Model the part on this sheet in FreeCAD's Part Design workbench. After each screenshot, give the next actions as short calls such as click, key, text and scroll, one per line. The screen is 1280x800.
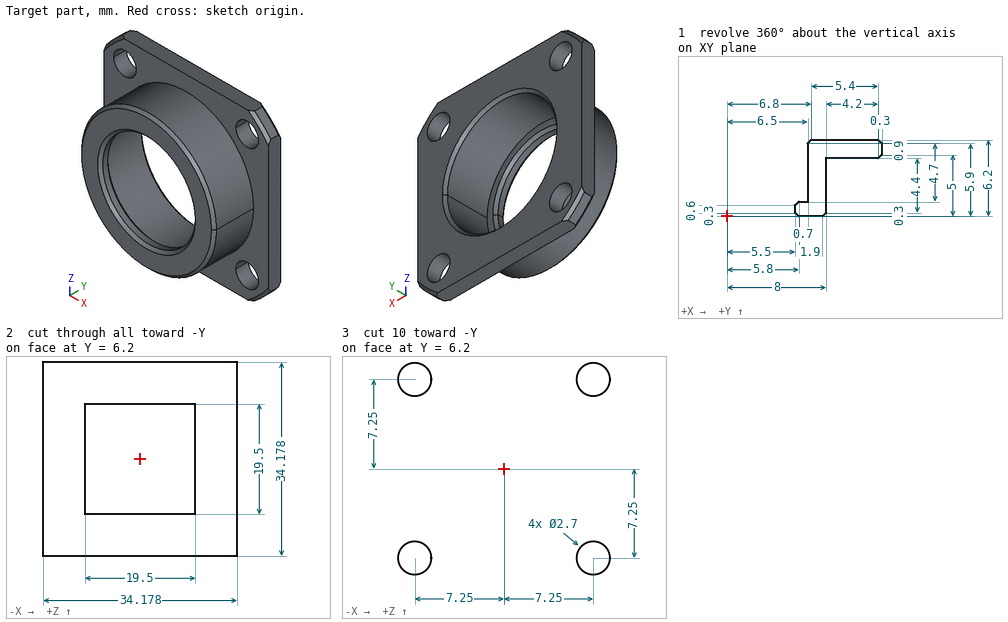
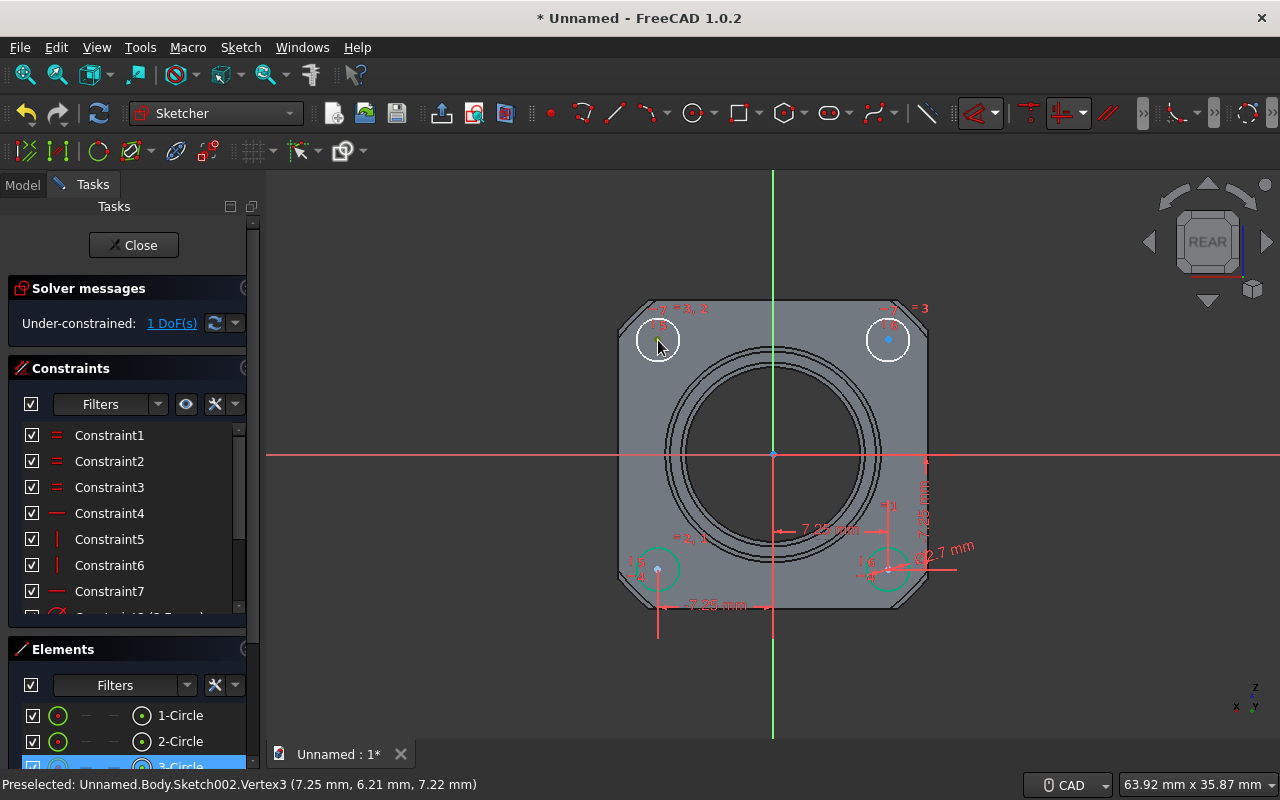
key(i)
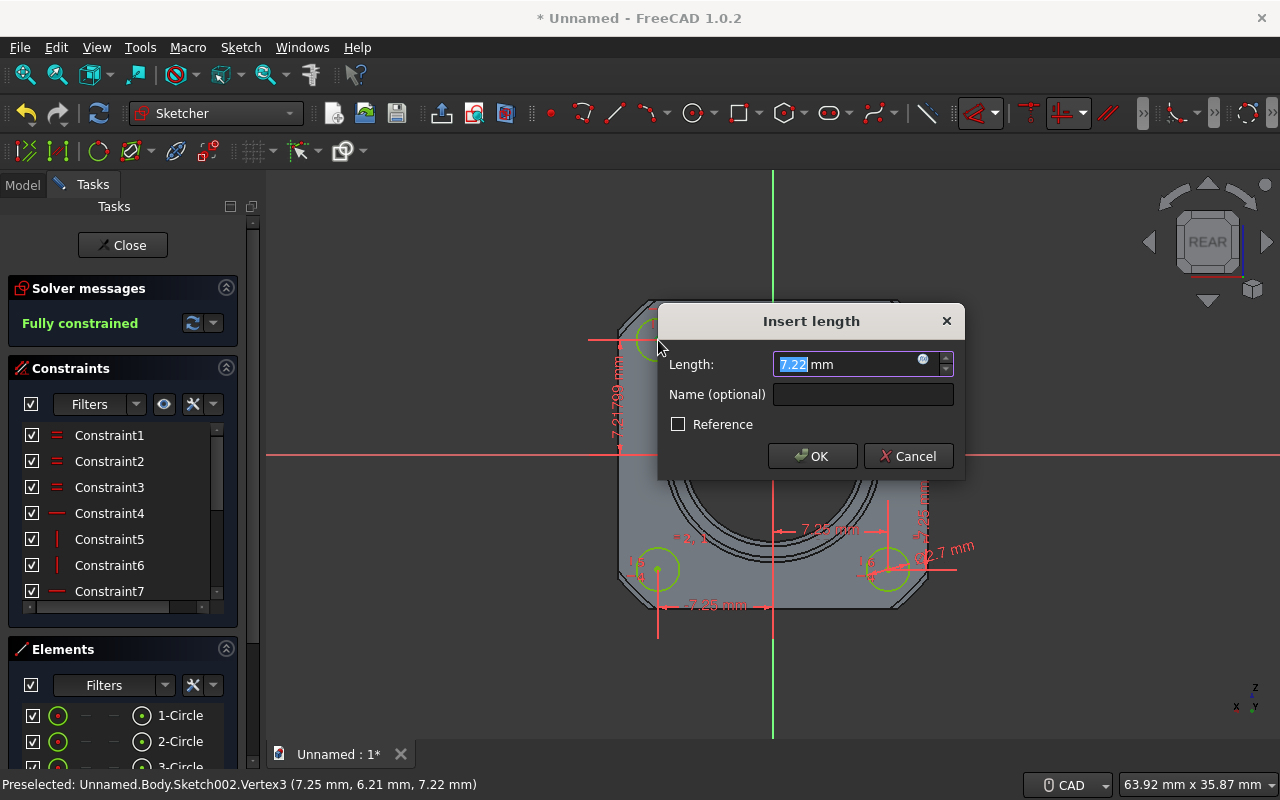
text(7.25)
key(Return)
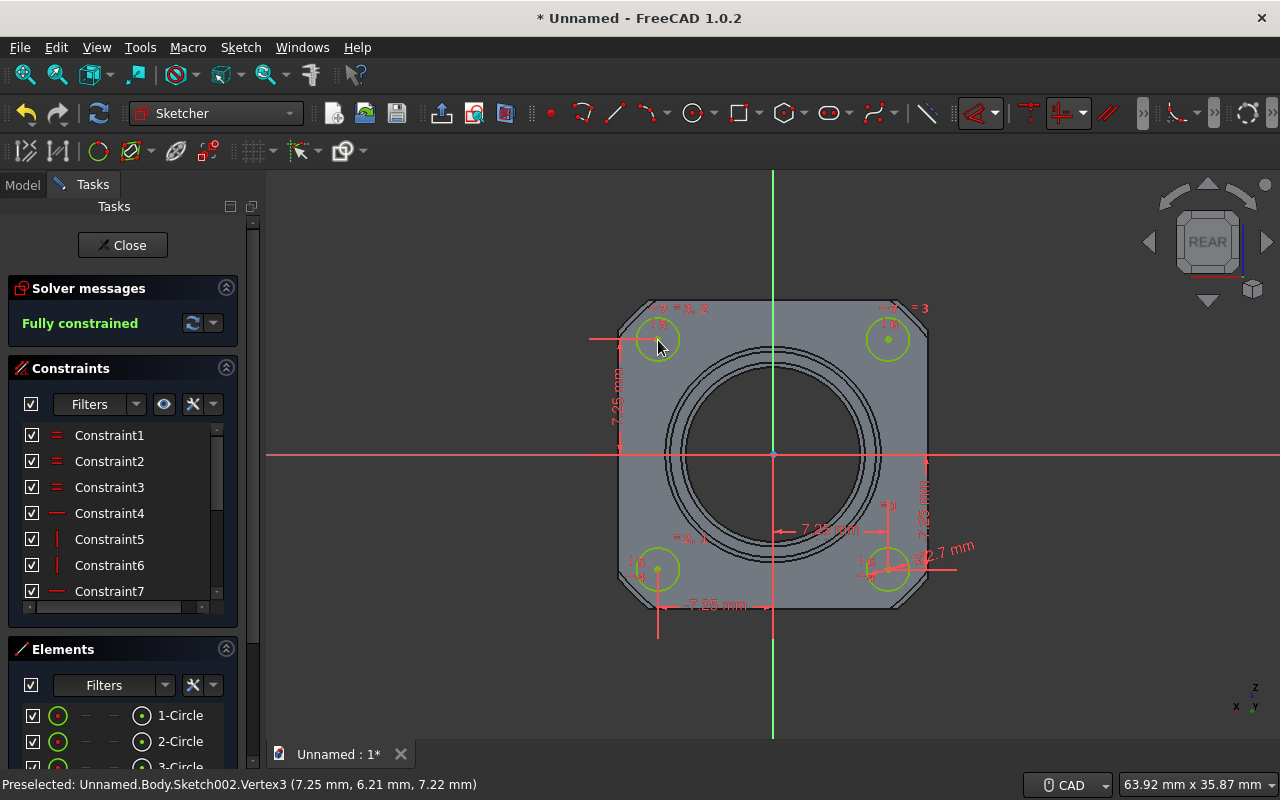
click(123, 245)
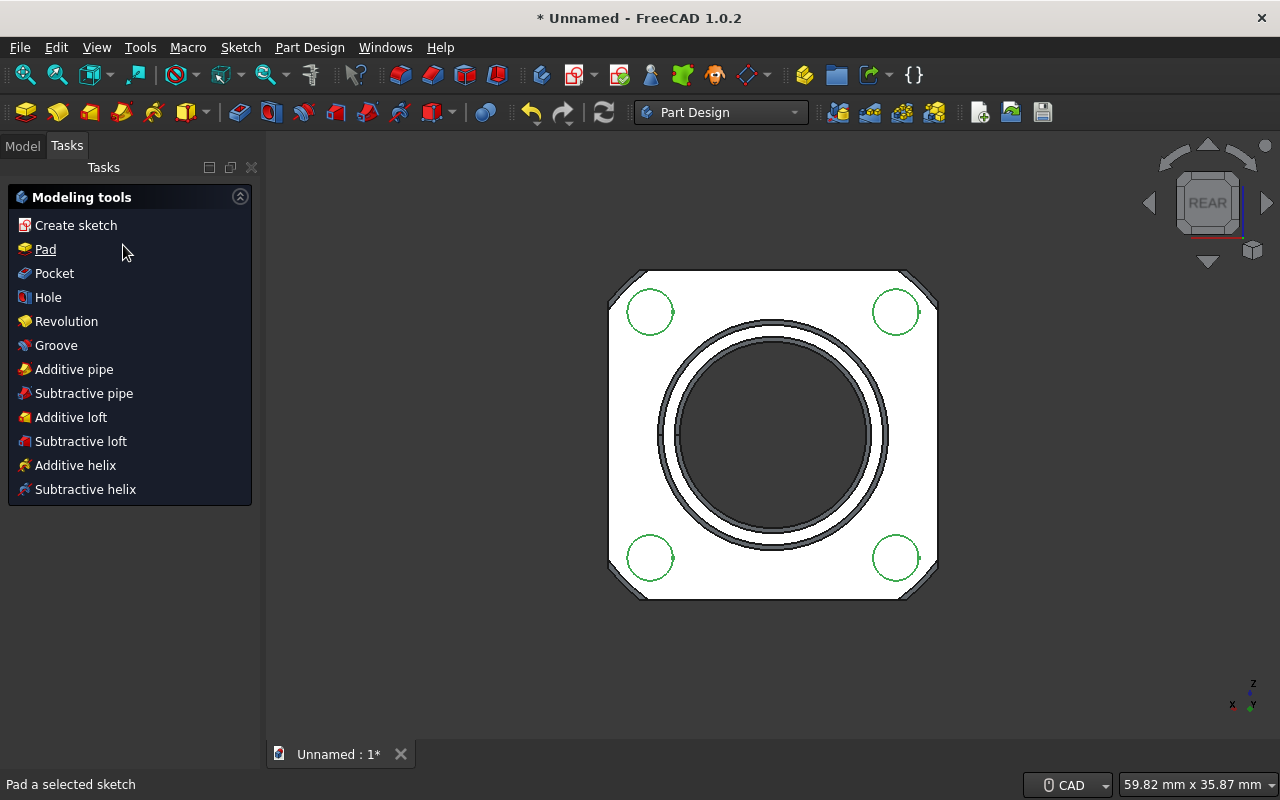
click(240, 112)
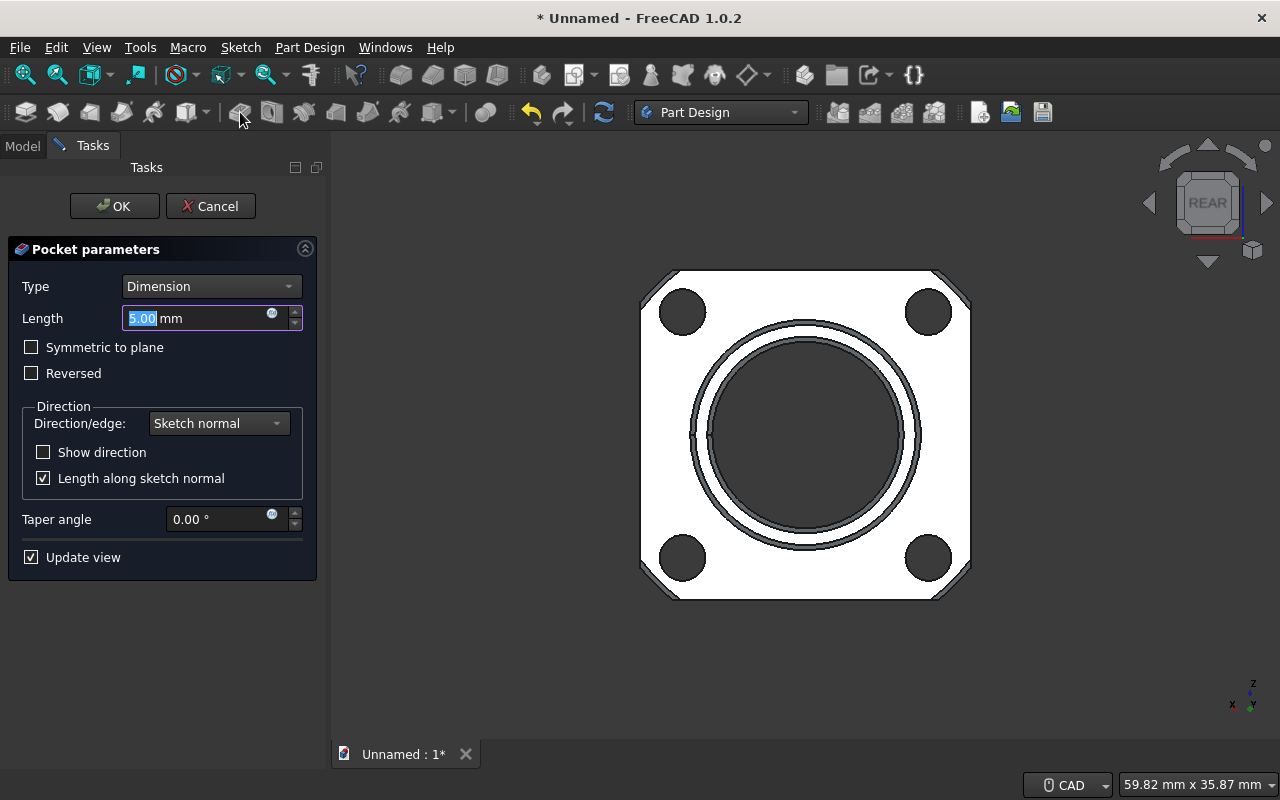
text(10)
key(Tab)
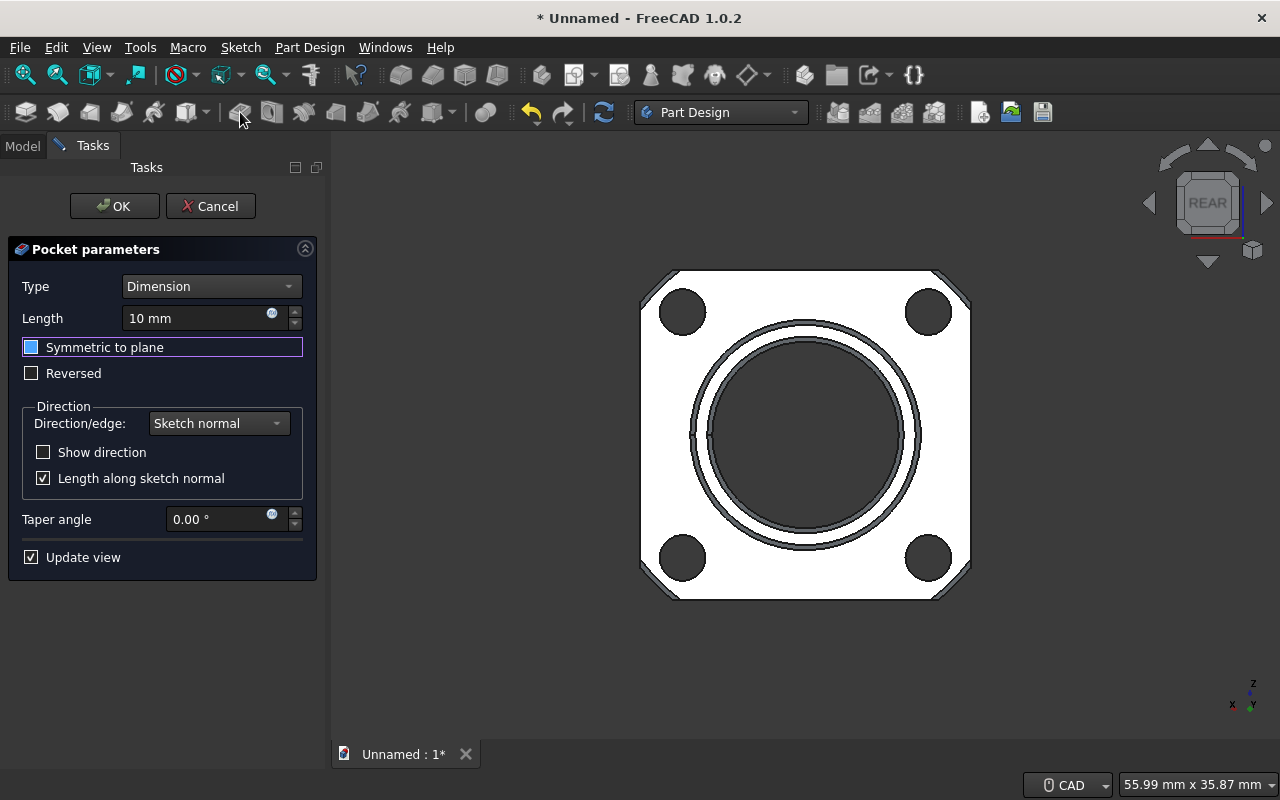
click(115, 206)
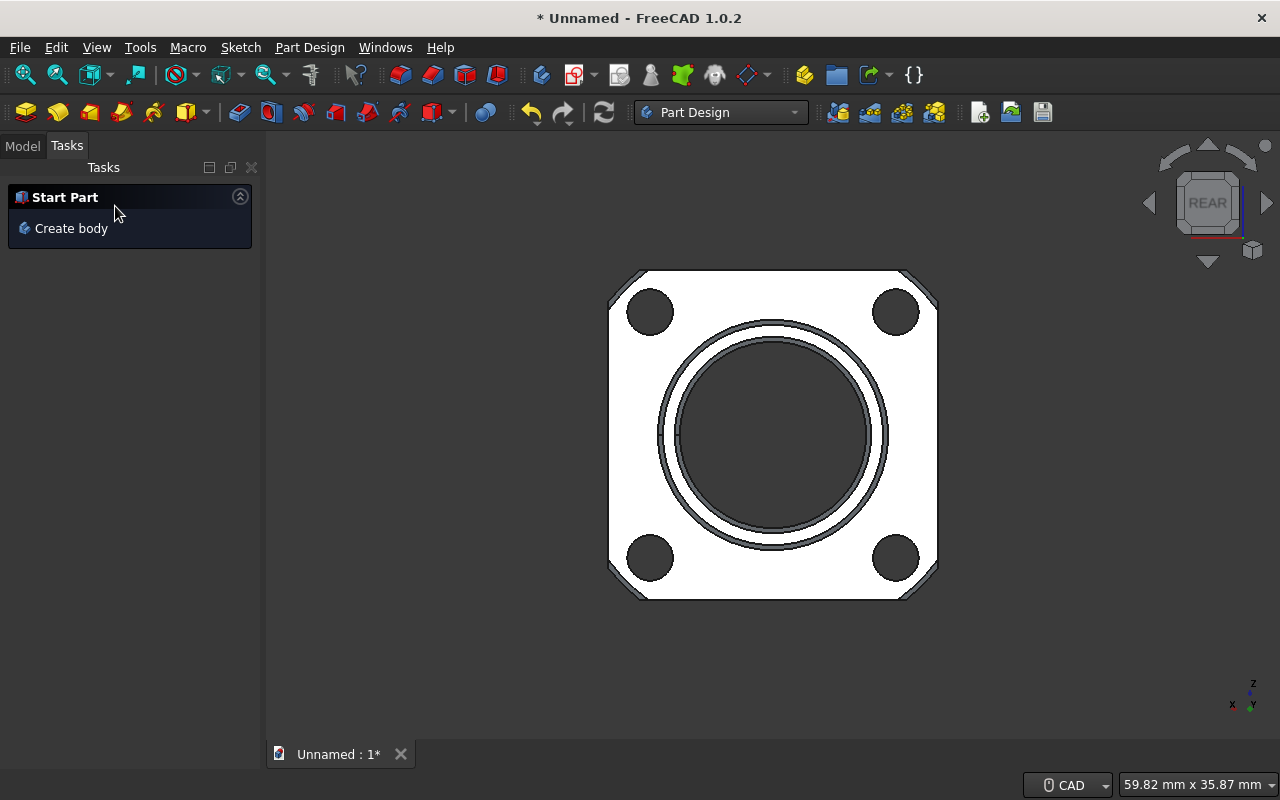
key(0)